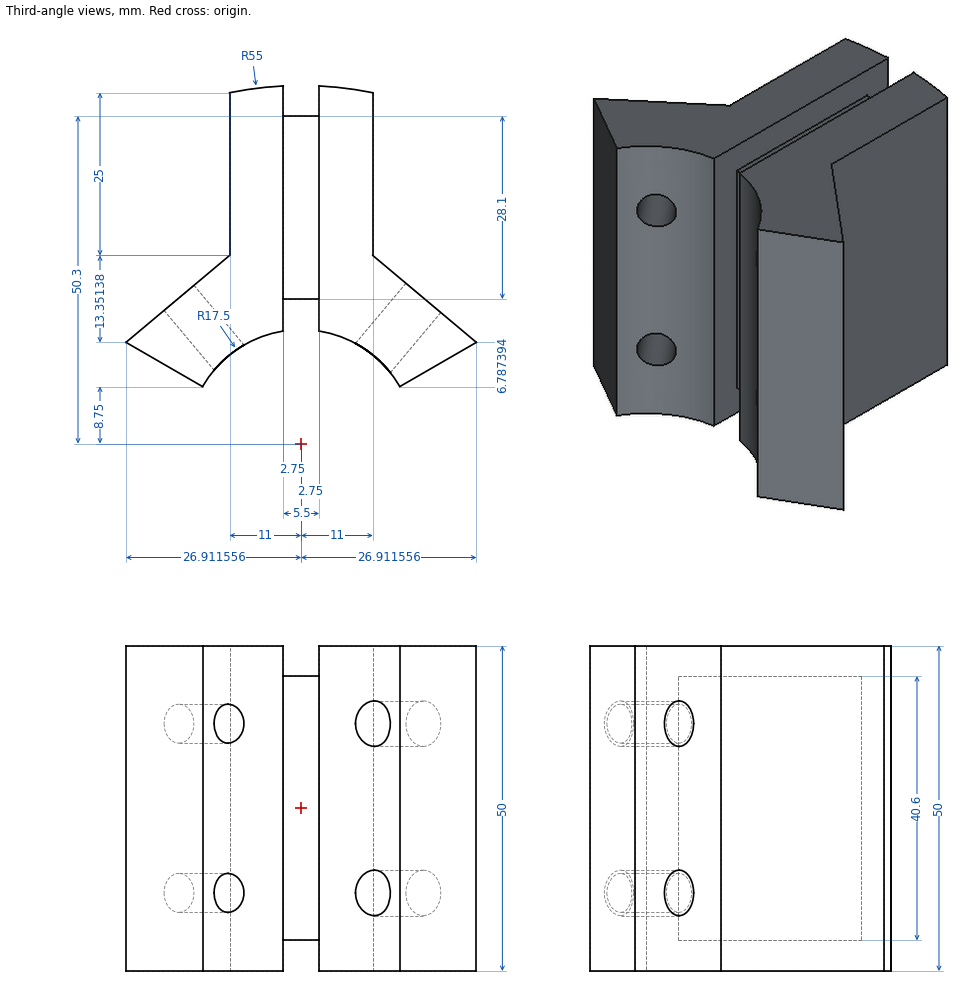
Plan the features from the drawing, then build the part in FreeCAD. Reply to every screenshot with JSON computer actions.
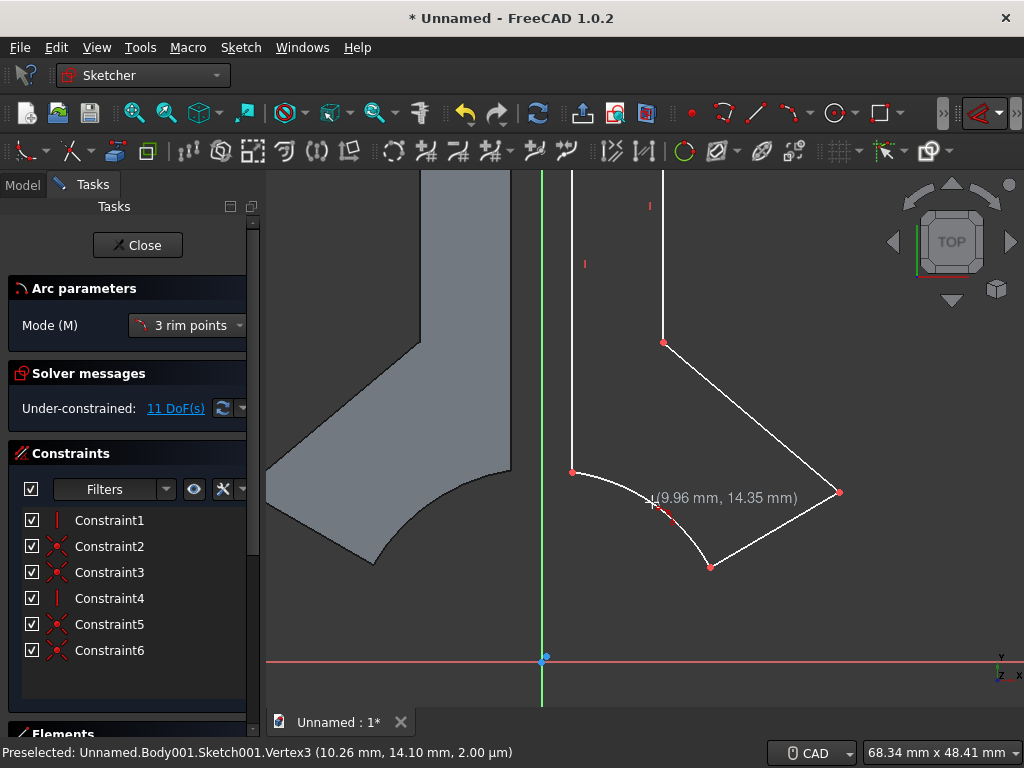
{"action": "scroll", "coordinate": [437, 537], "scroll_direction": "down", "scroll_amount": 3}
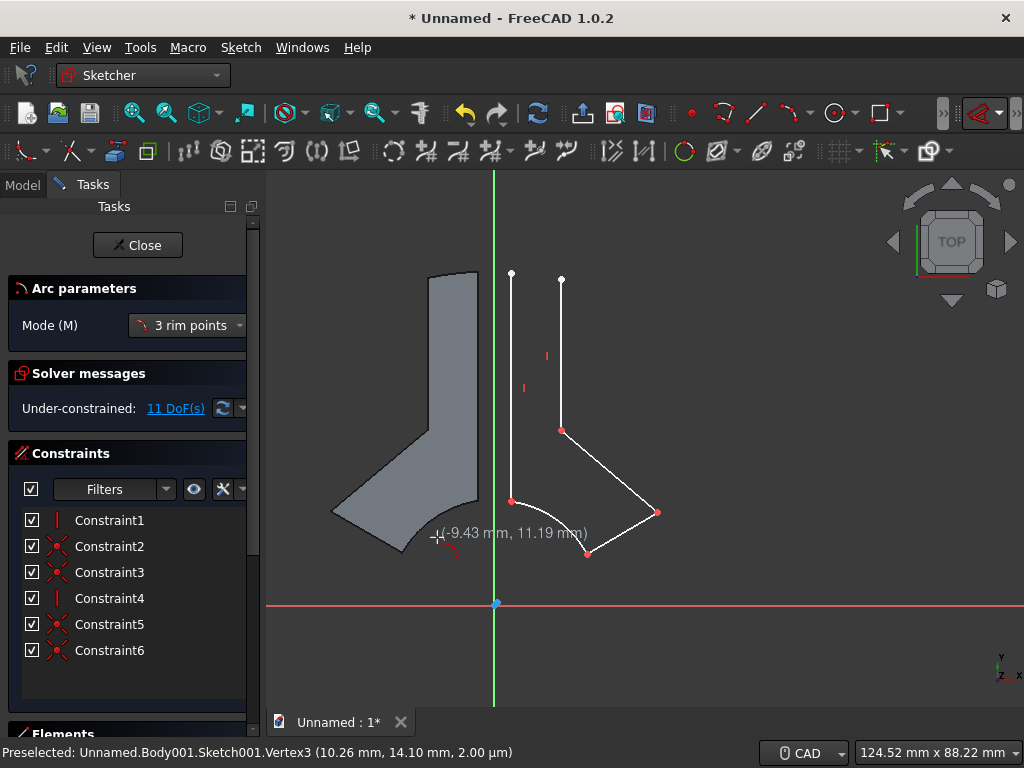
{"action": "left_click", "coordinate": [561, 279]}
{"action": "left_click", "coordinate": [511, 273]}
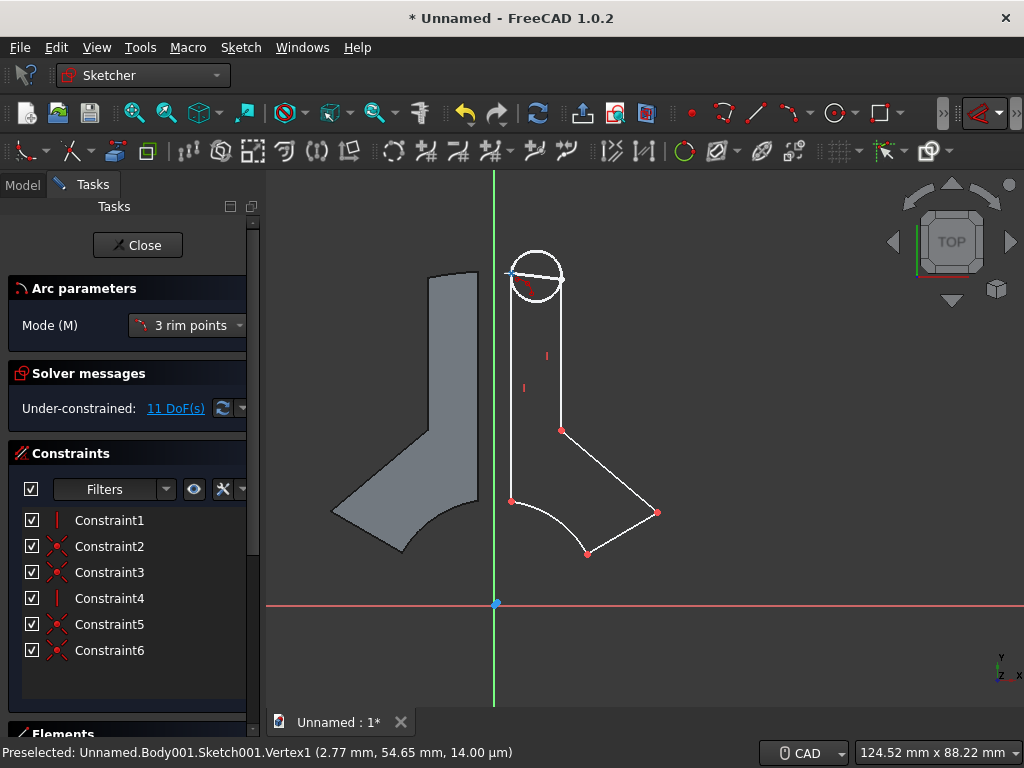
{"action": "scroll", "coordinate": [536, 274], "scroll_direction": "up", "scroll_amount": 15}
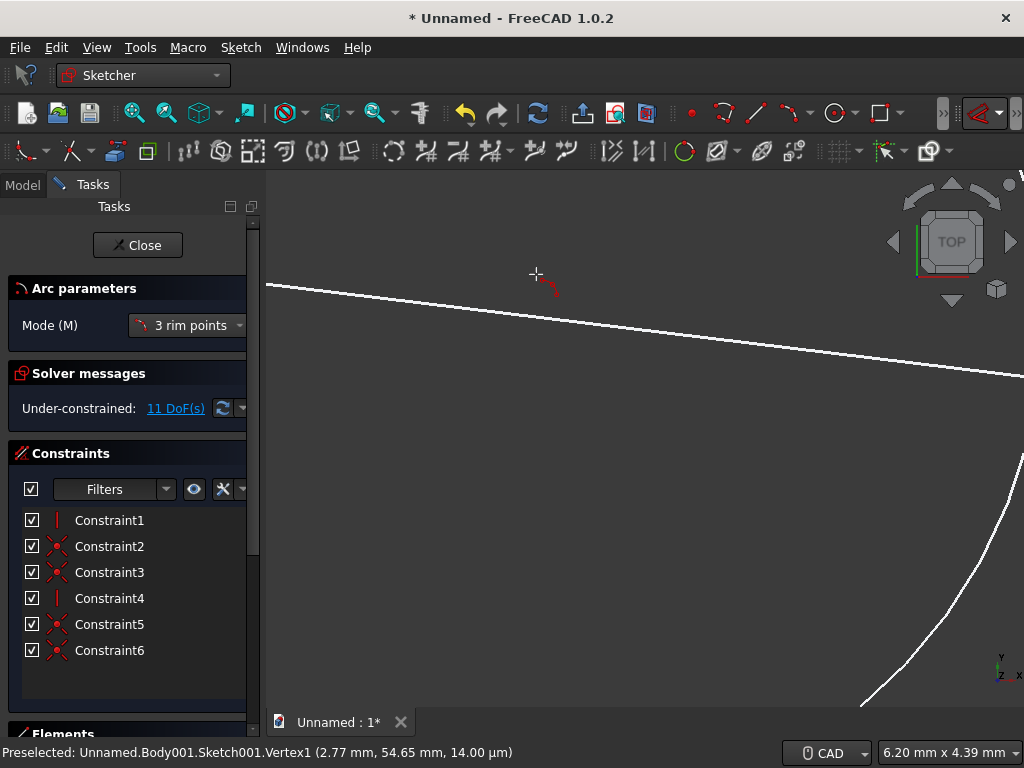
{"action": "left_click", "coordinate": [538, 267]}
{"action": "key", "text": "Escape"}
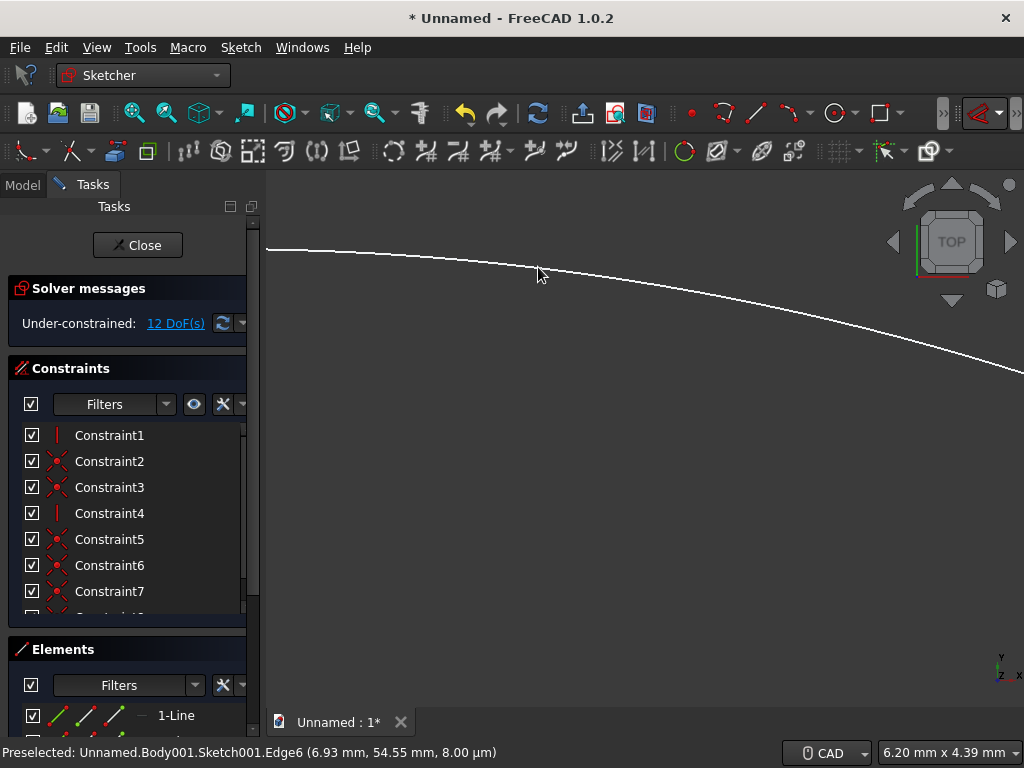
{"action": "scroll", "coordinate": [536, 274], "scroll_direction": "down", "scroll_amount": 15}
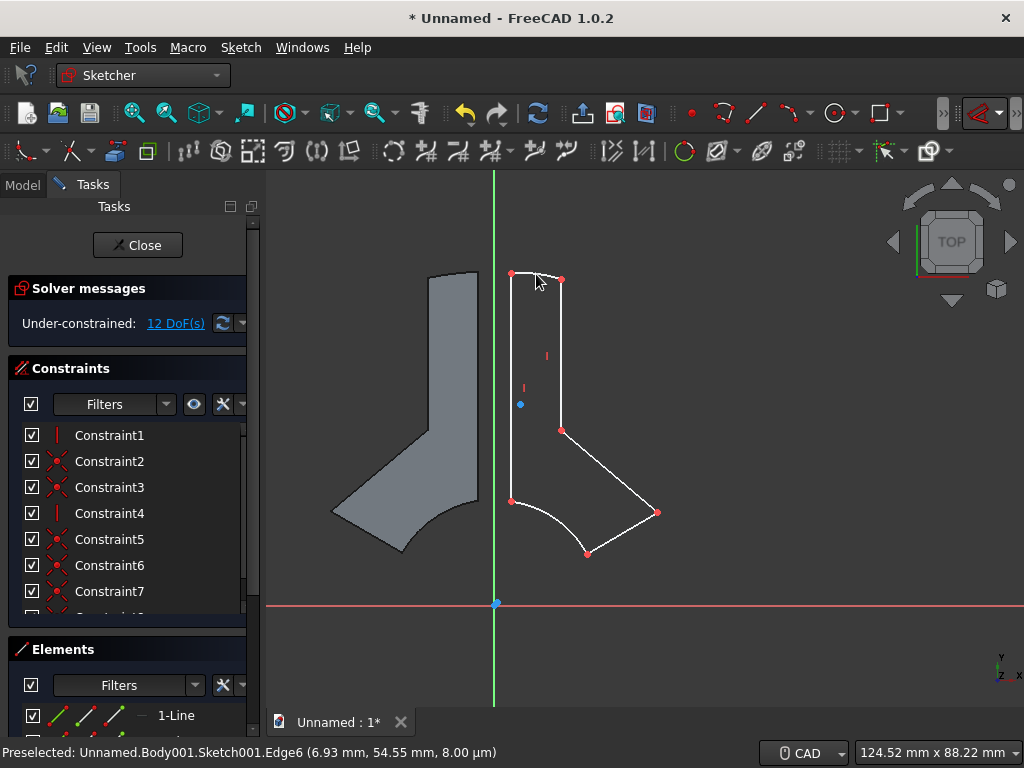
{"action": "left_click", "coordinate": [570, 531]}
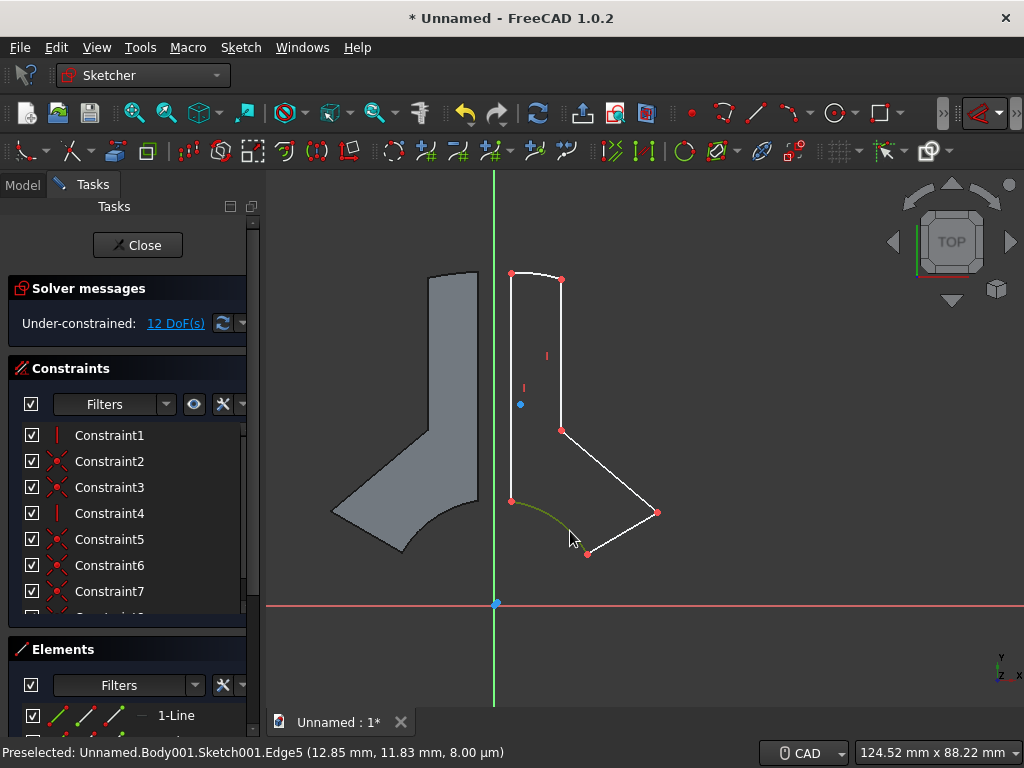
{"action": "left_click", "coordinate": [547, 276]}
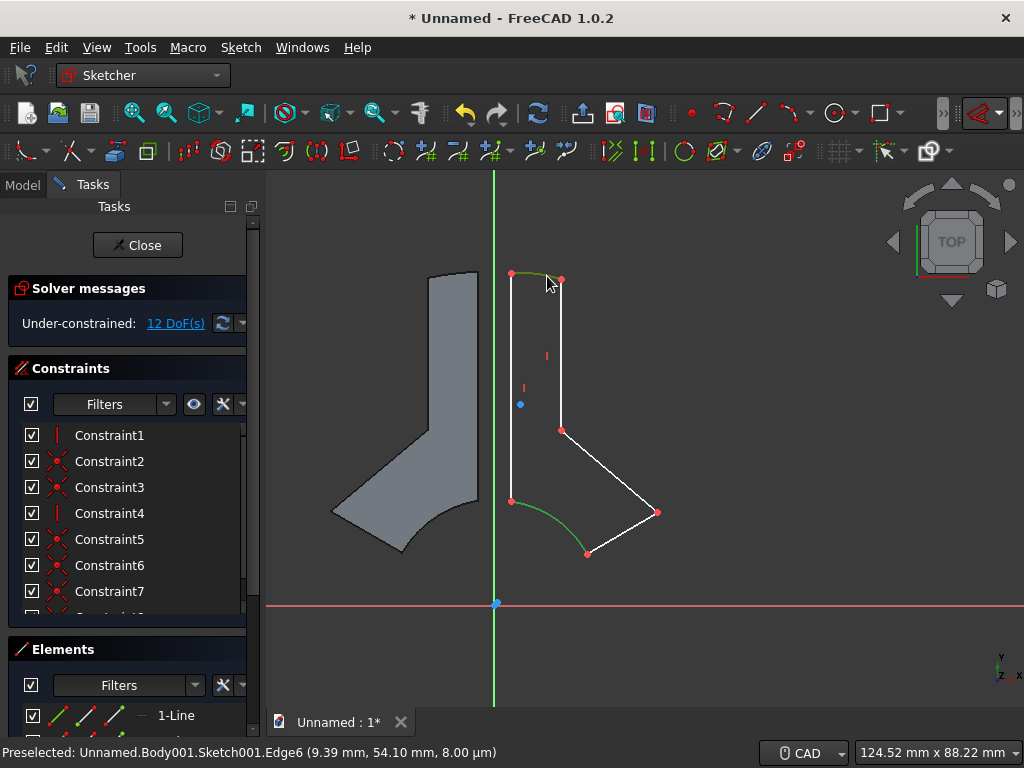
{"action": "key", "text": "c"}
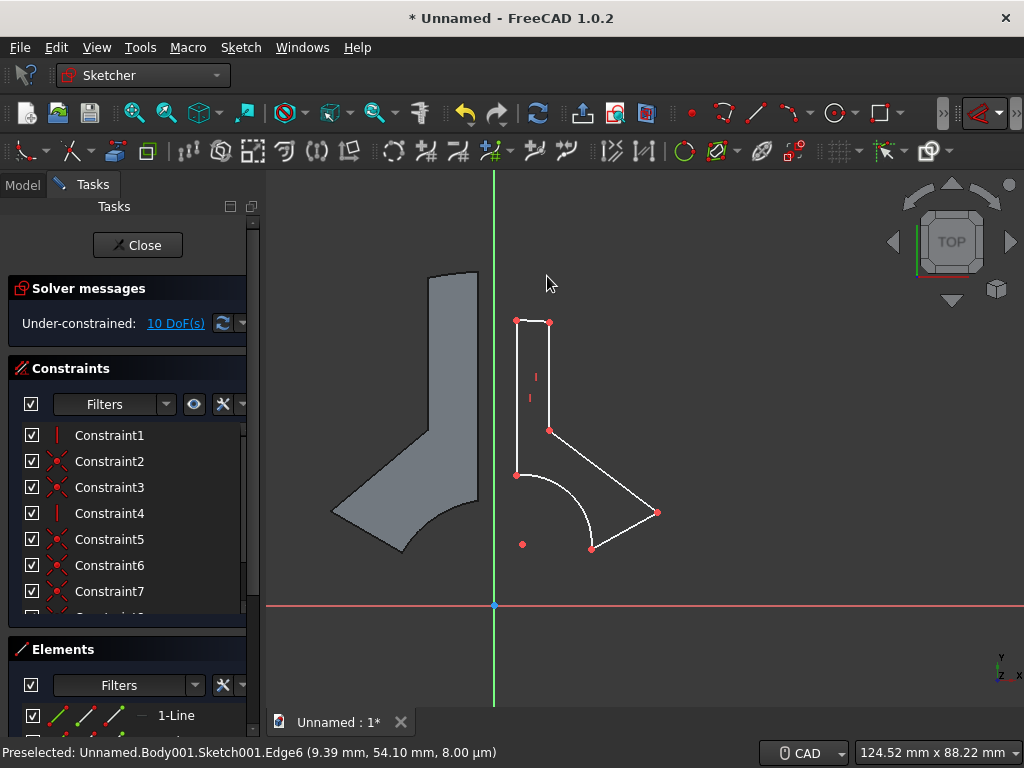
{"action": "left_click_drag", "start_coordinate": [484, 534], "coordinate": [532, 616]}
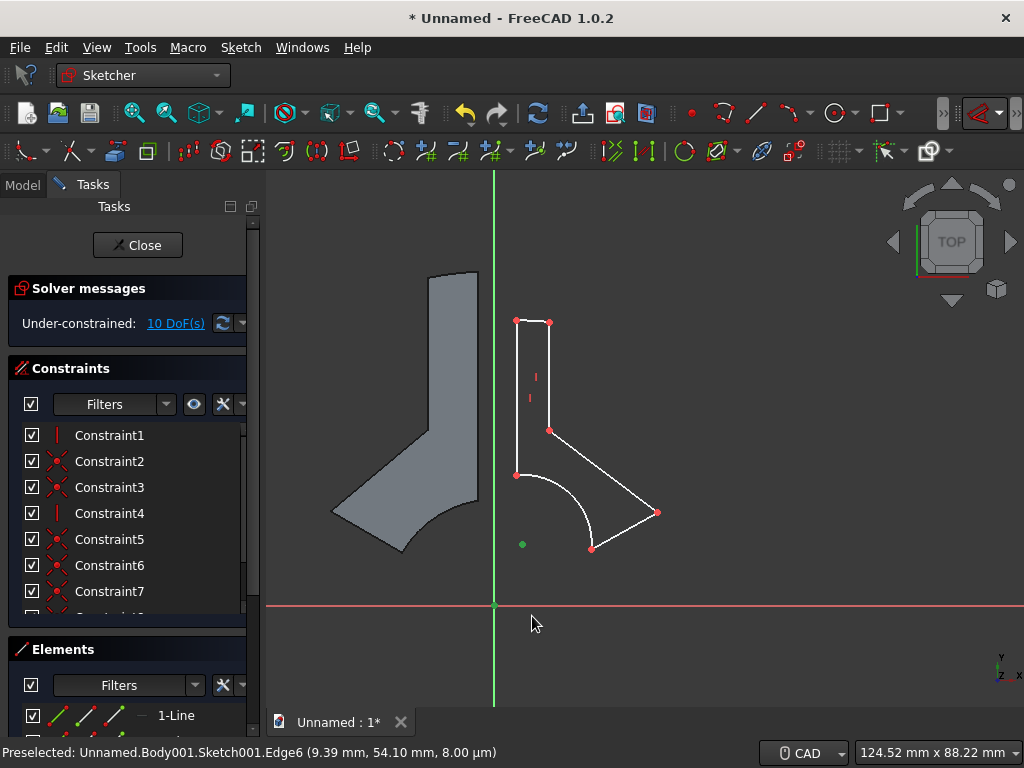
{"action": "key", "text": "c"}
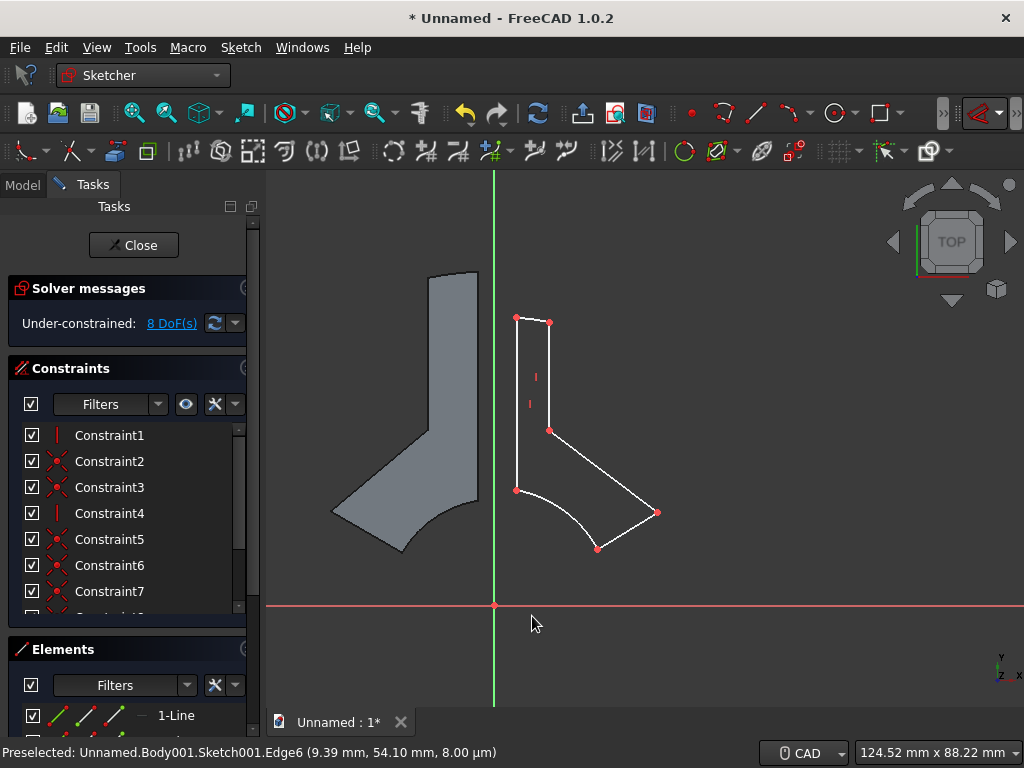
{"action": "left_click", "coordinate": [580, 524]}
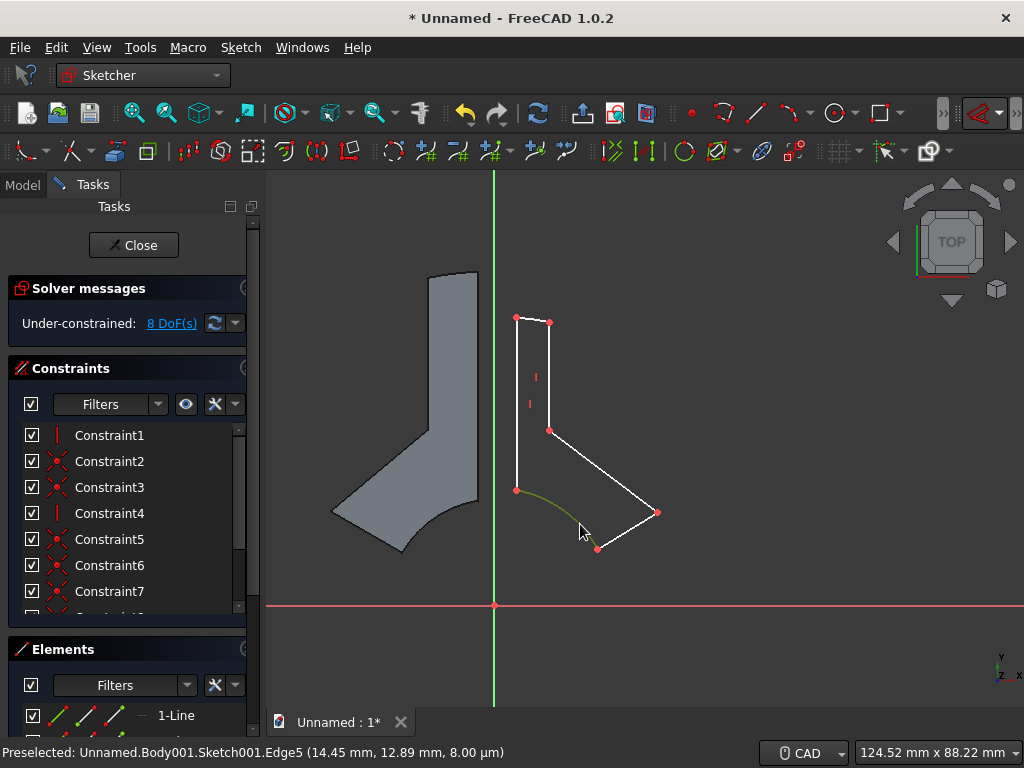
{"action": "key", "text": "k r"}